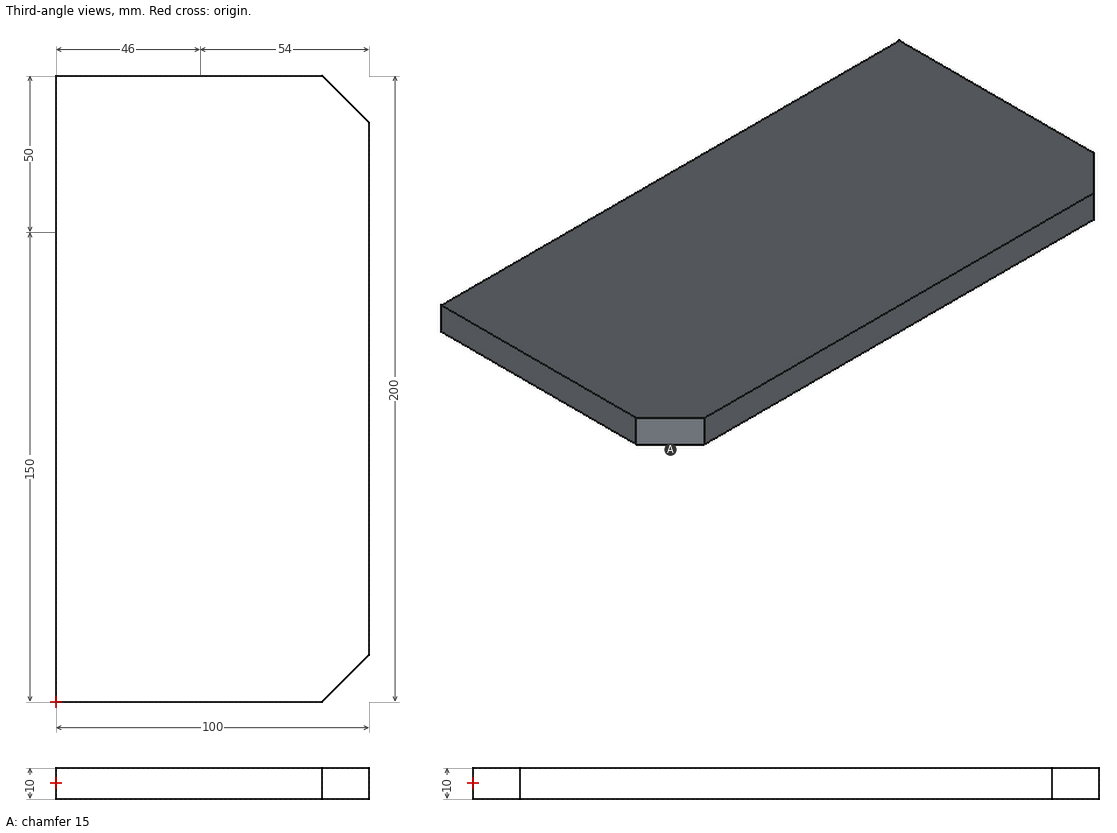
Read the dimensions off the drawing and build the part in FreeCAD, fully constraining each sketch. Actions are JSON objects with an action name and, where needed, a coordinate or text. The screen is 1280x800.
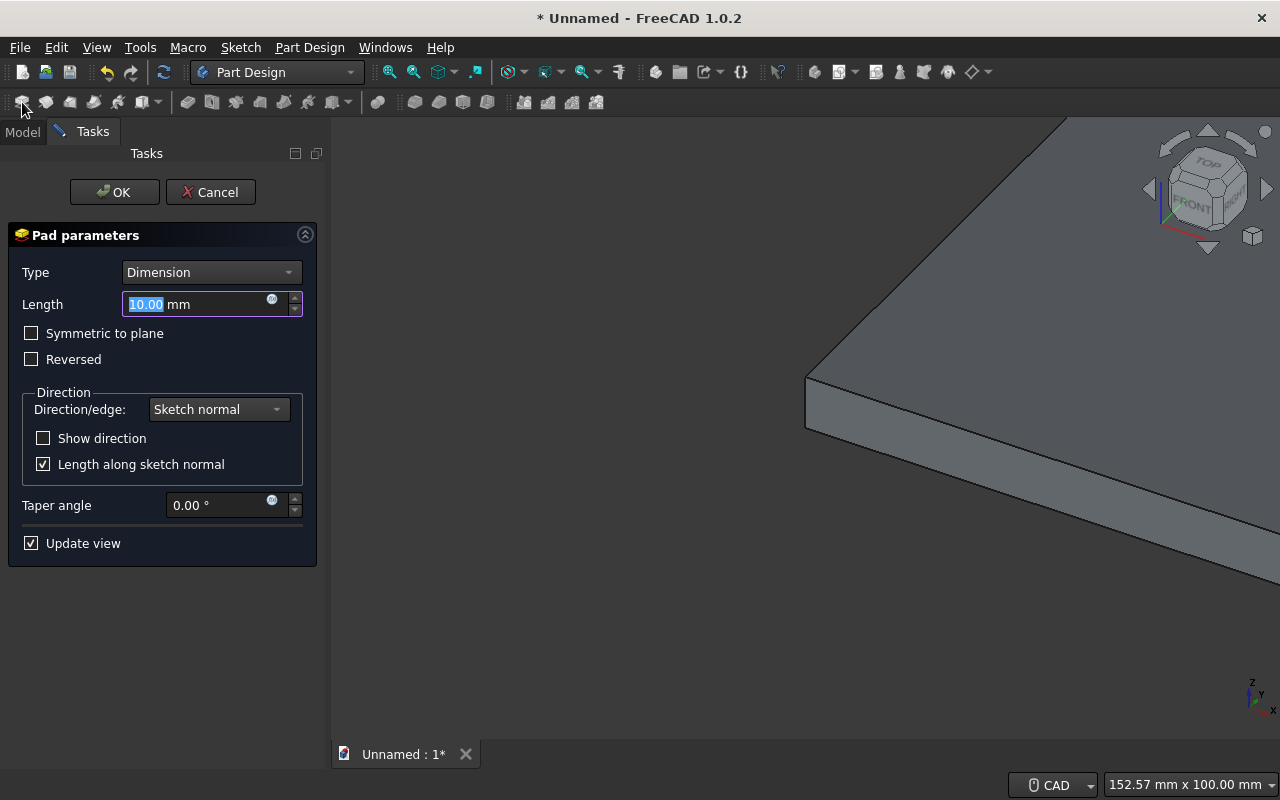
{"action": "type", "text": "10"}
{"action": "key", "text": "Tab"}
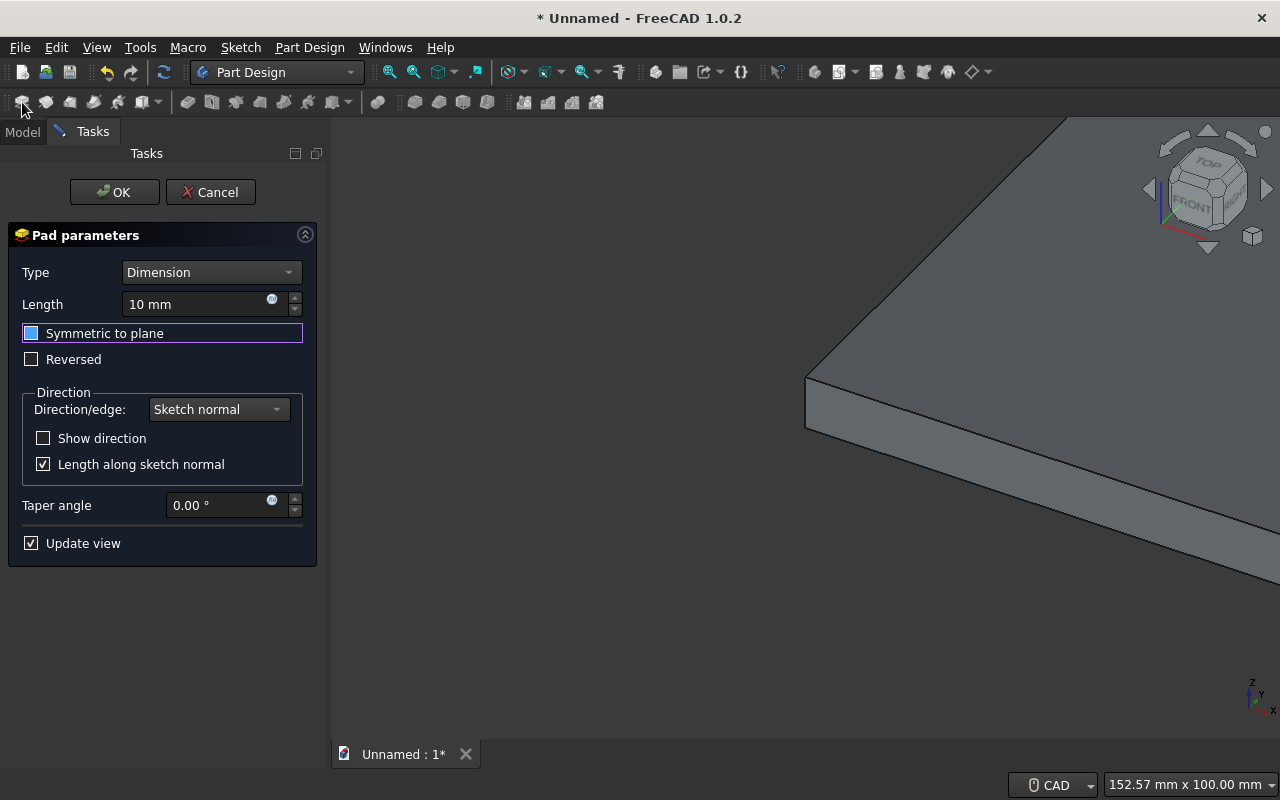
{"action": "left_click", "coordinate": [30, 333]}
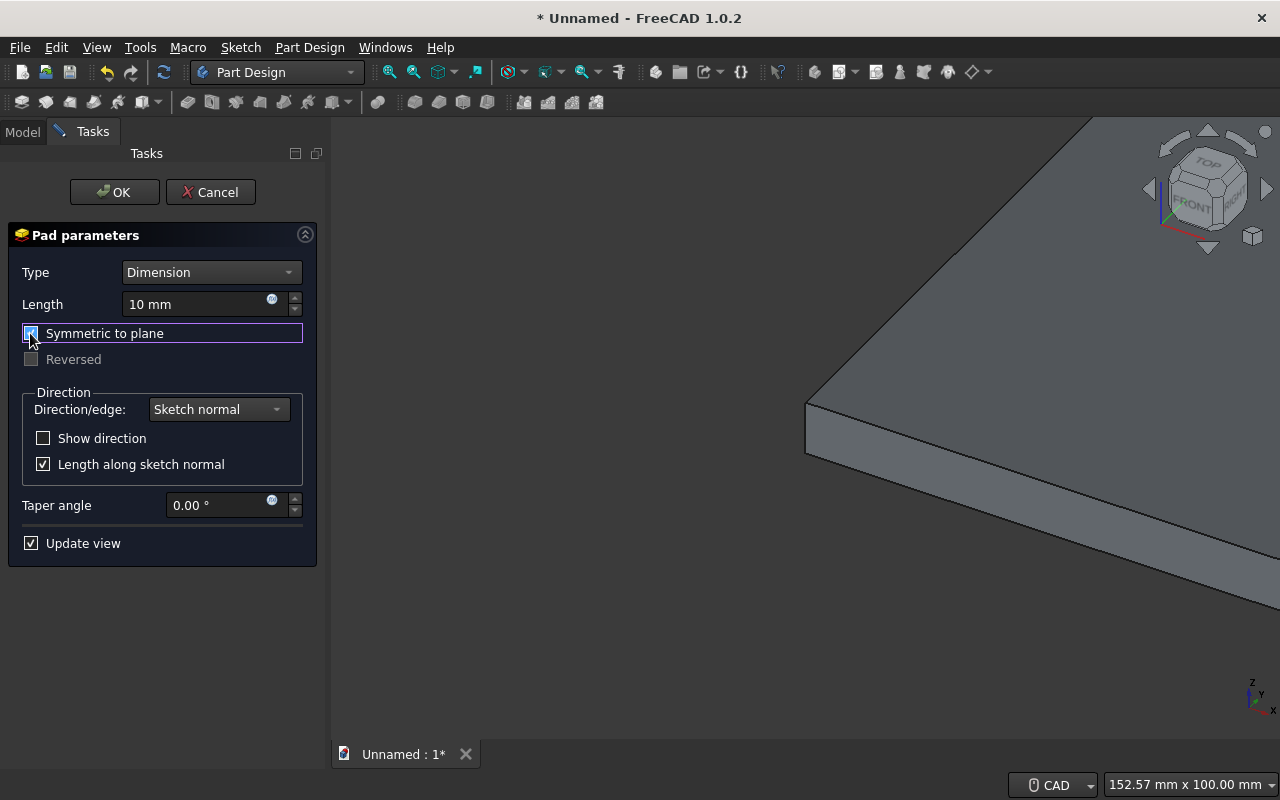
{"action": "left_click", "coordinate": [115, 192]}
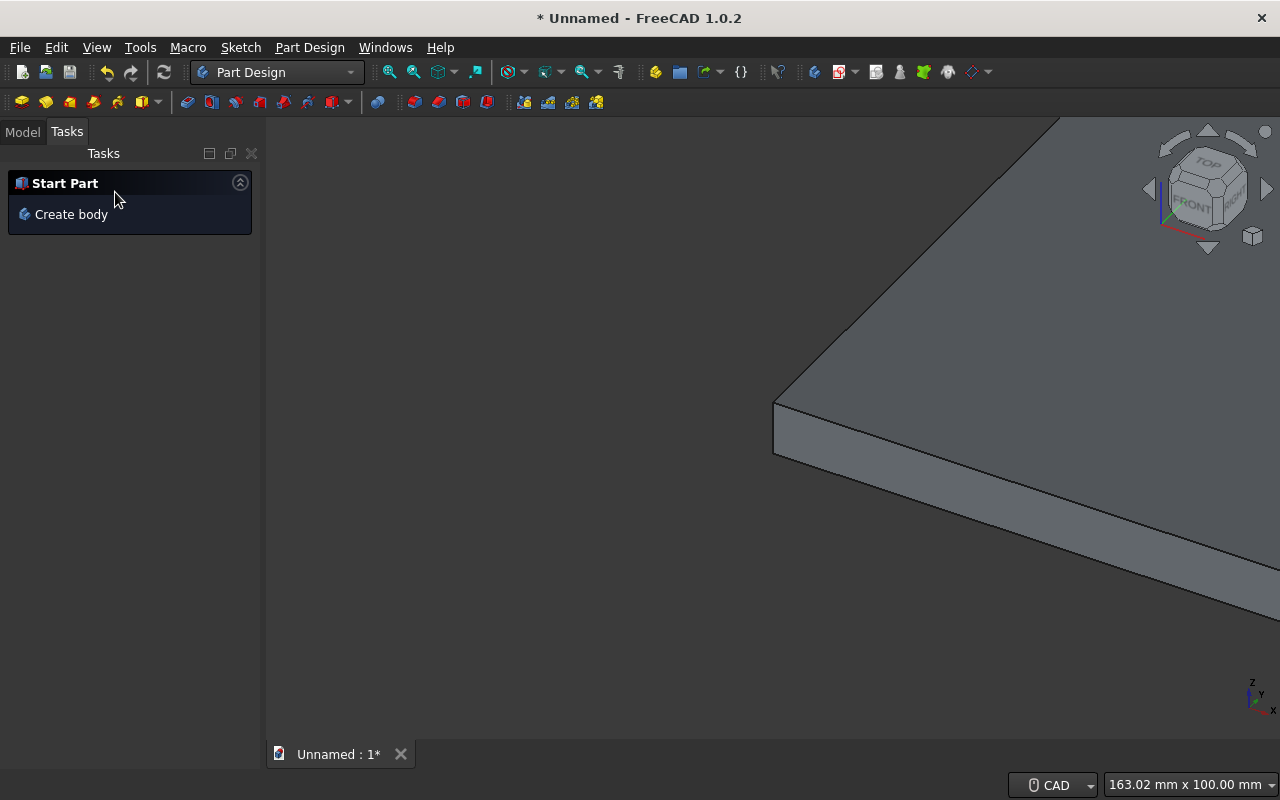
{"action": "left_click", "coordinate": [390, 72]}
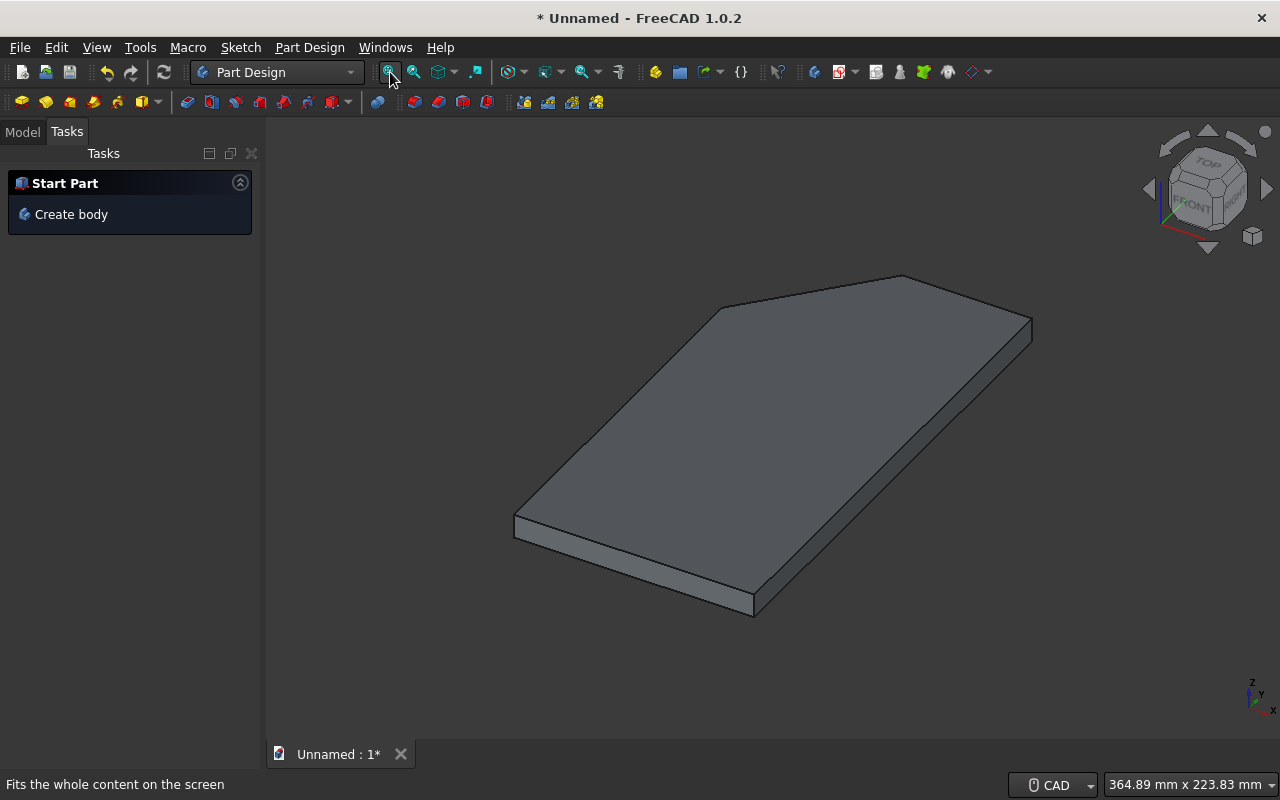
{"action": "left_click", "coordinate": [754, 605]}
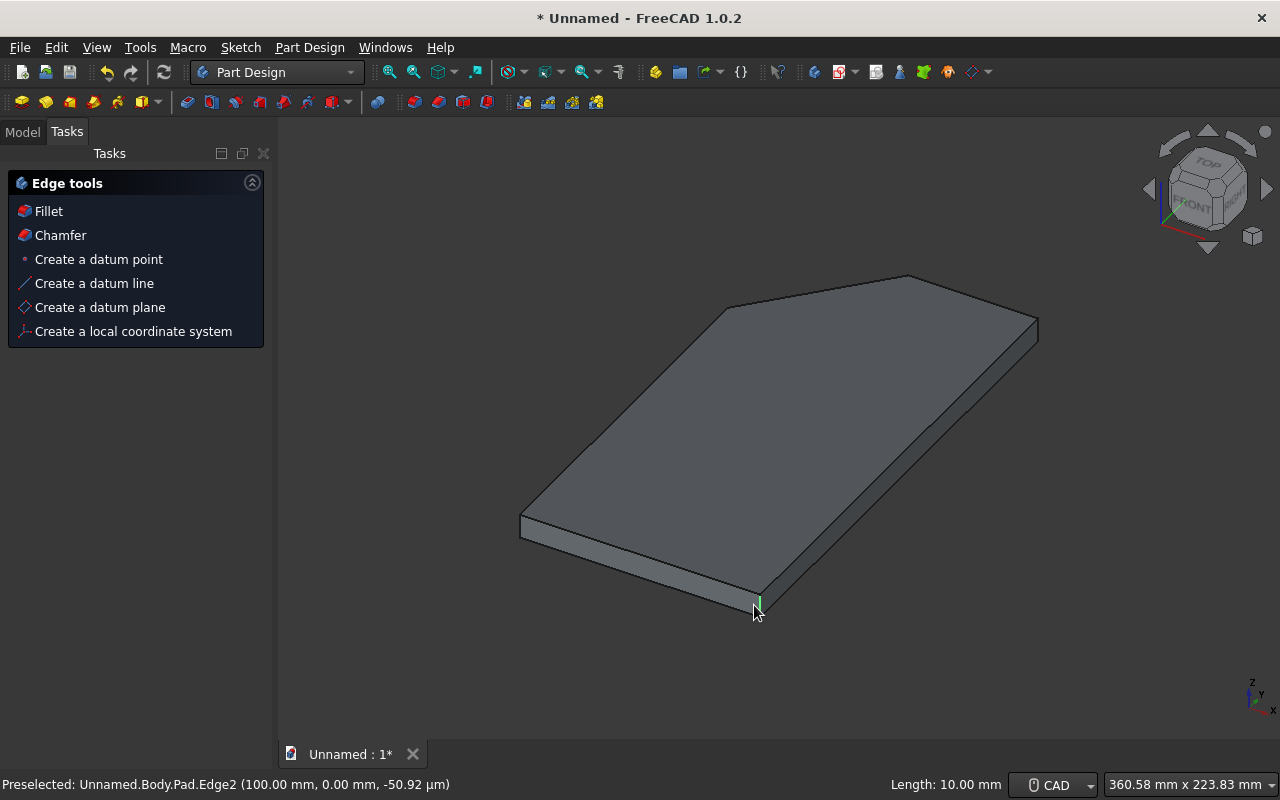
{"action": "key", "text": "0"}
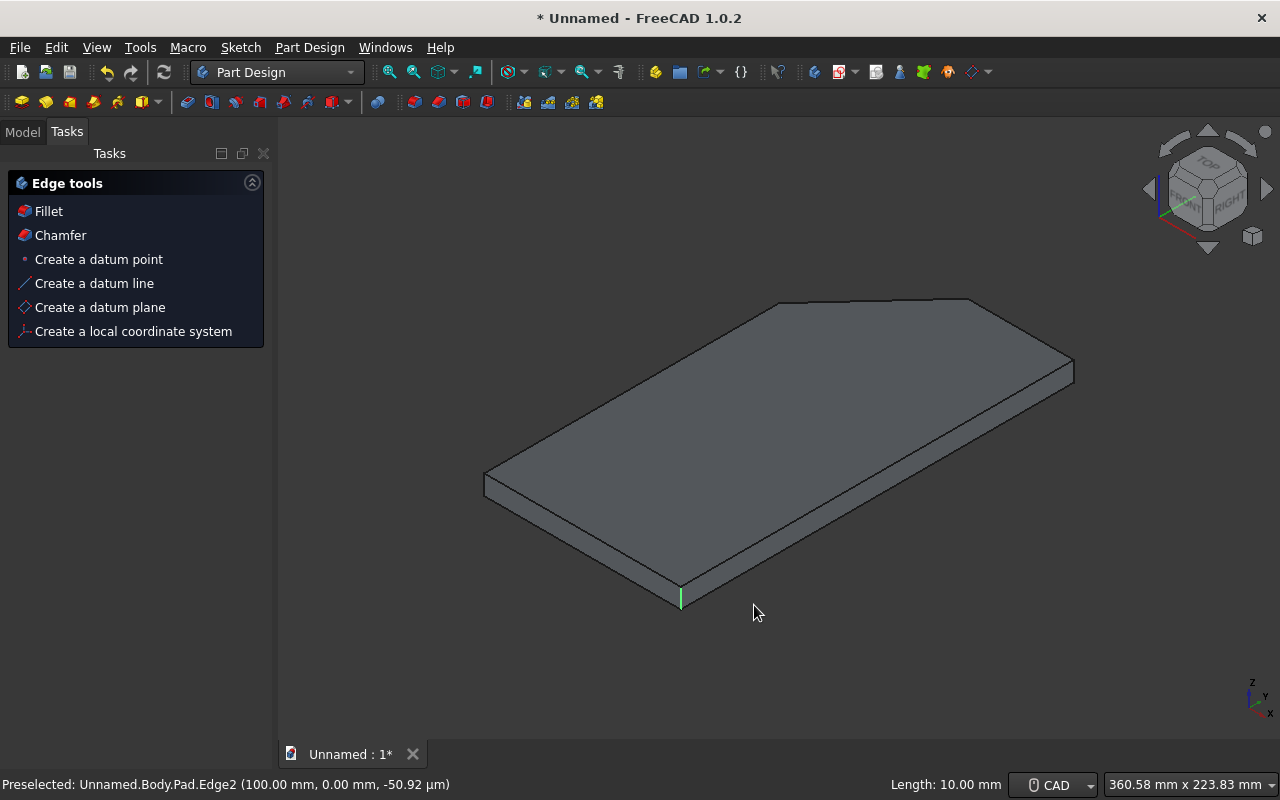
{"action": "key", "text": "2"}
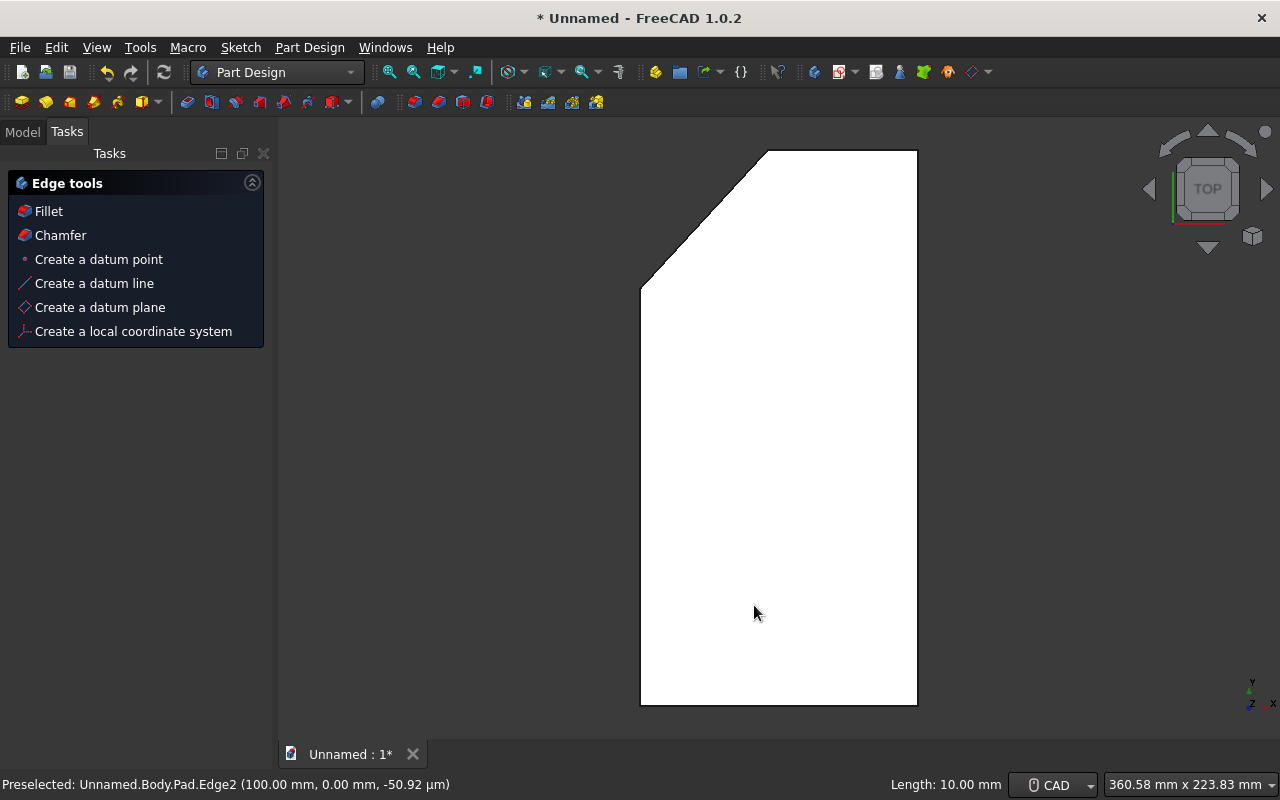
{"action": "key", "text": "1"}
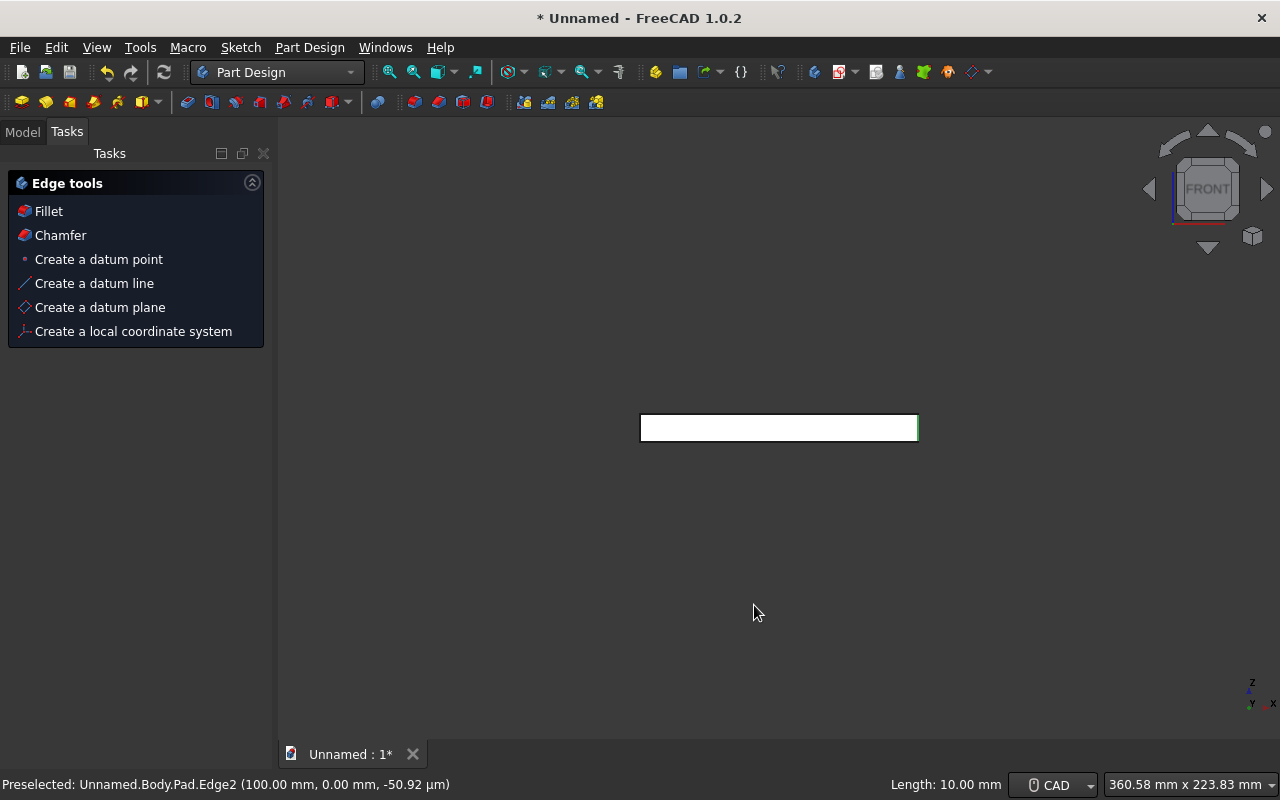
{"action": "key", "text": "v f"}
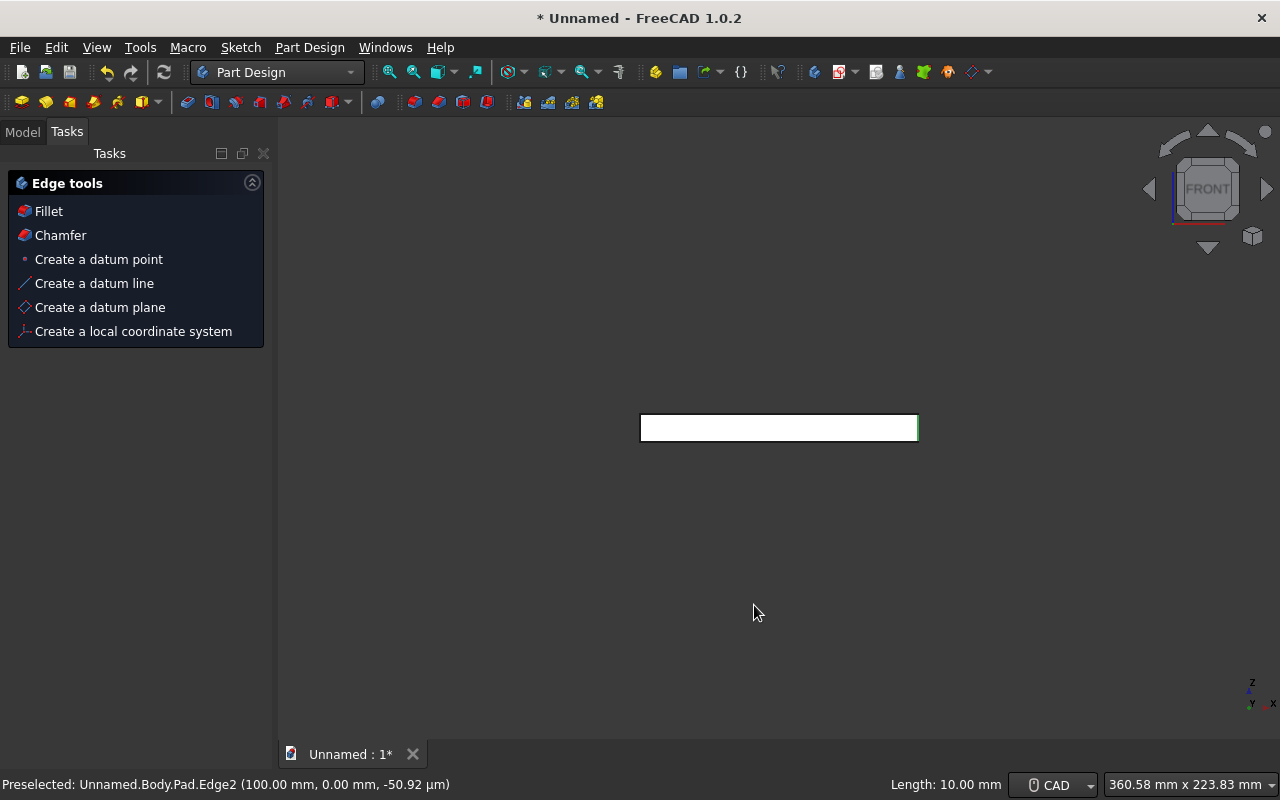
{"action": "key", "text": "3"}